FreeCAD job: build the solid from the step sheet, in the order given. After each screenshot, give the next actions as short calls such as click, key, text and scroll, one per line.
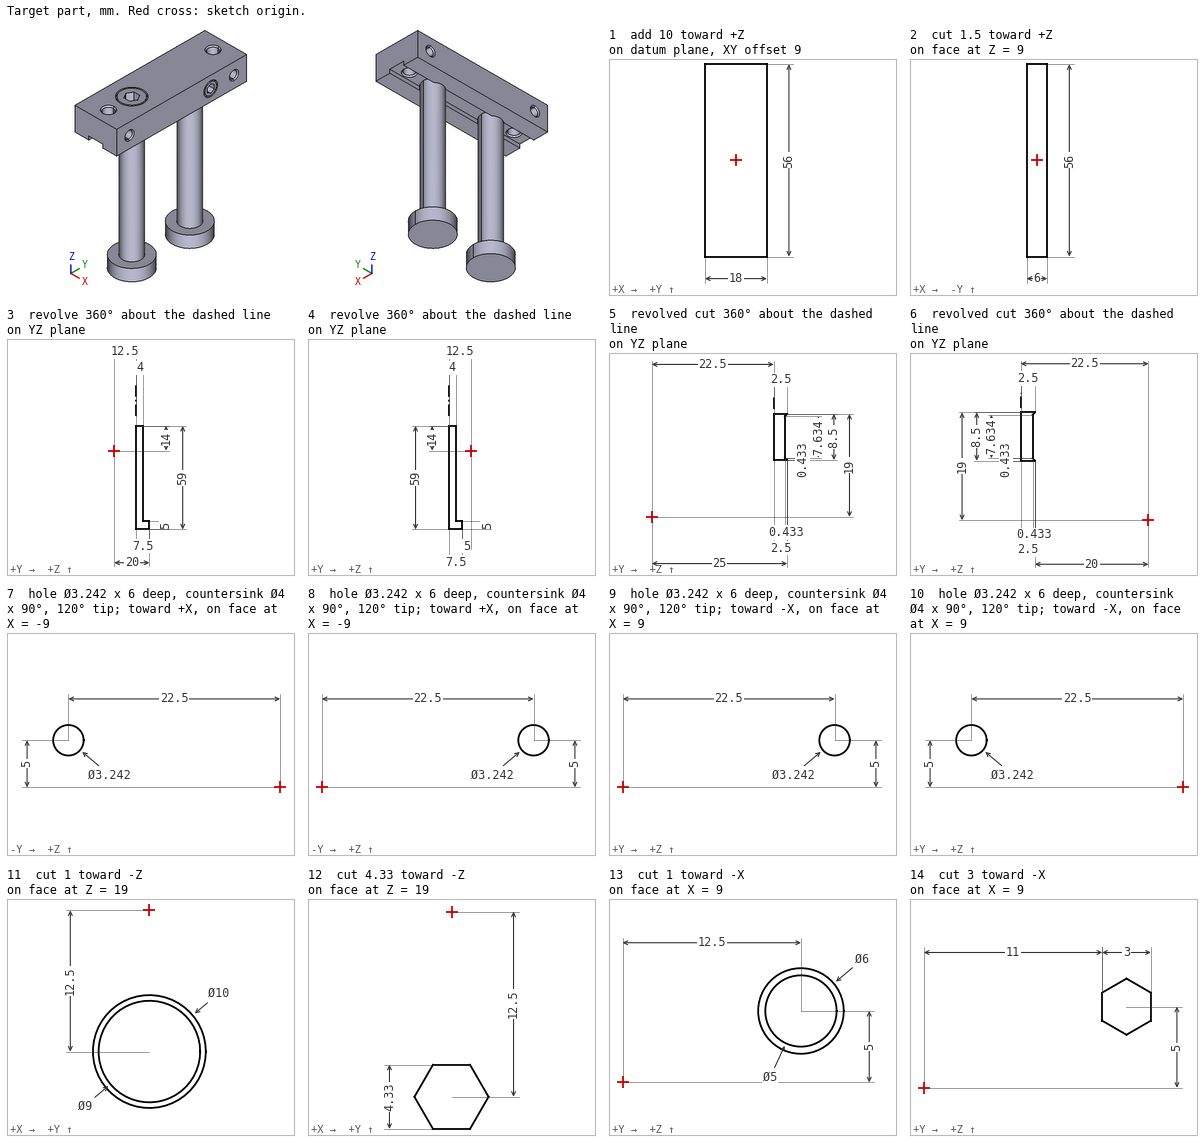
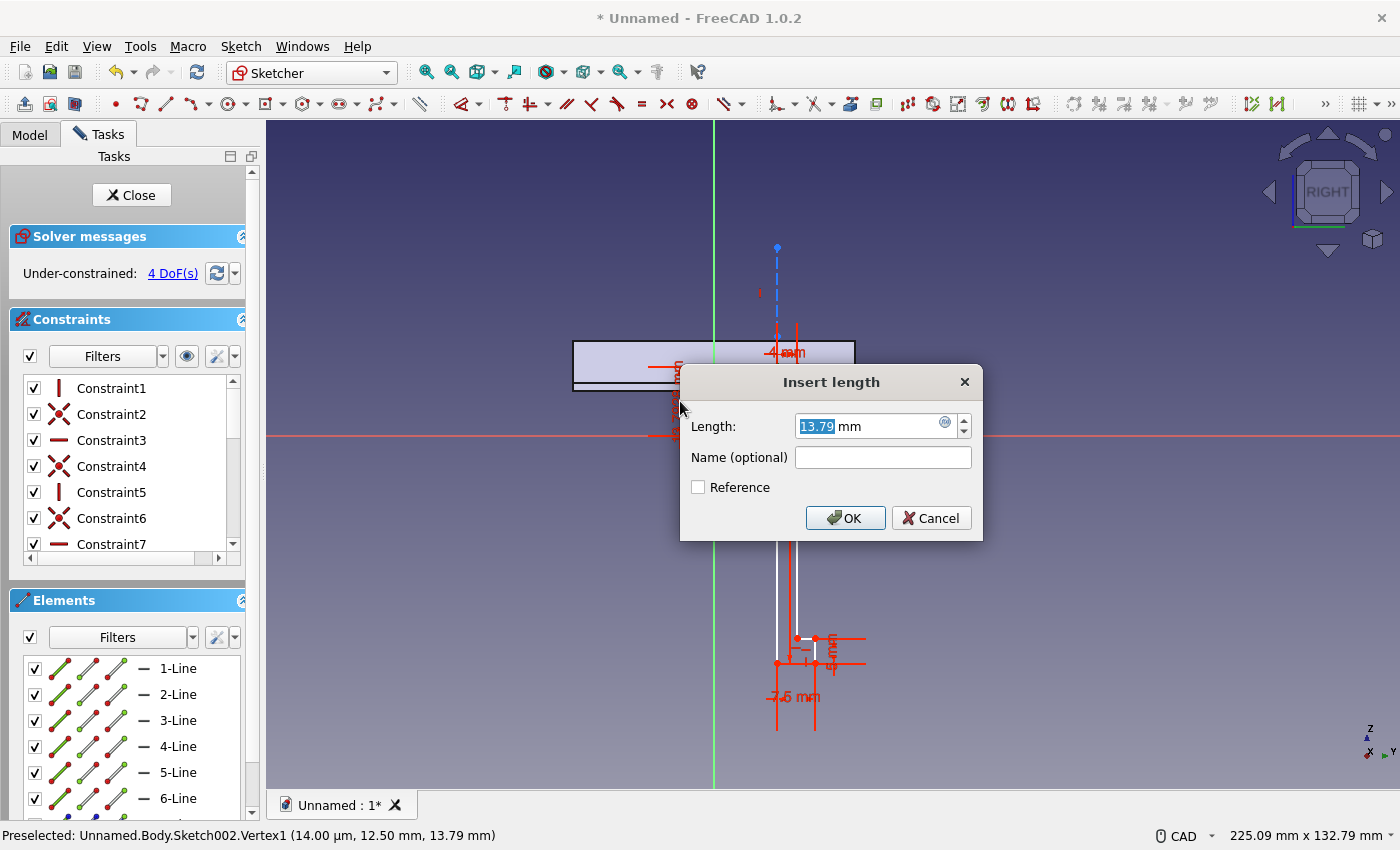
text(14)
key(Return)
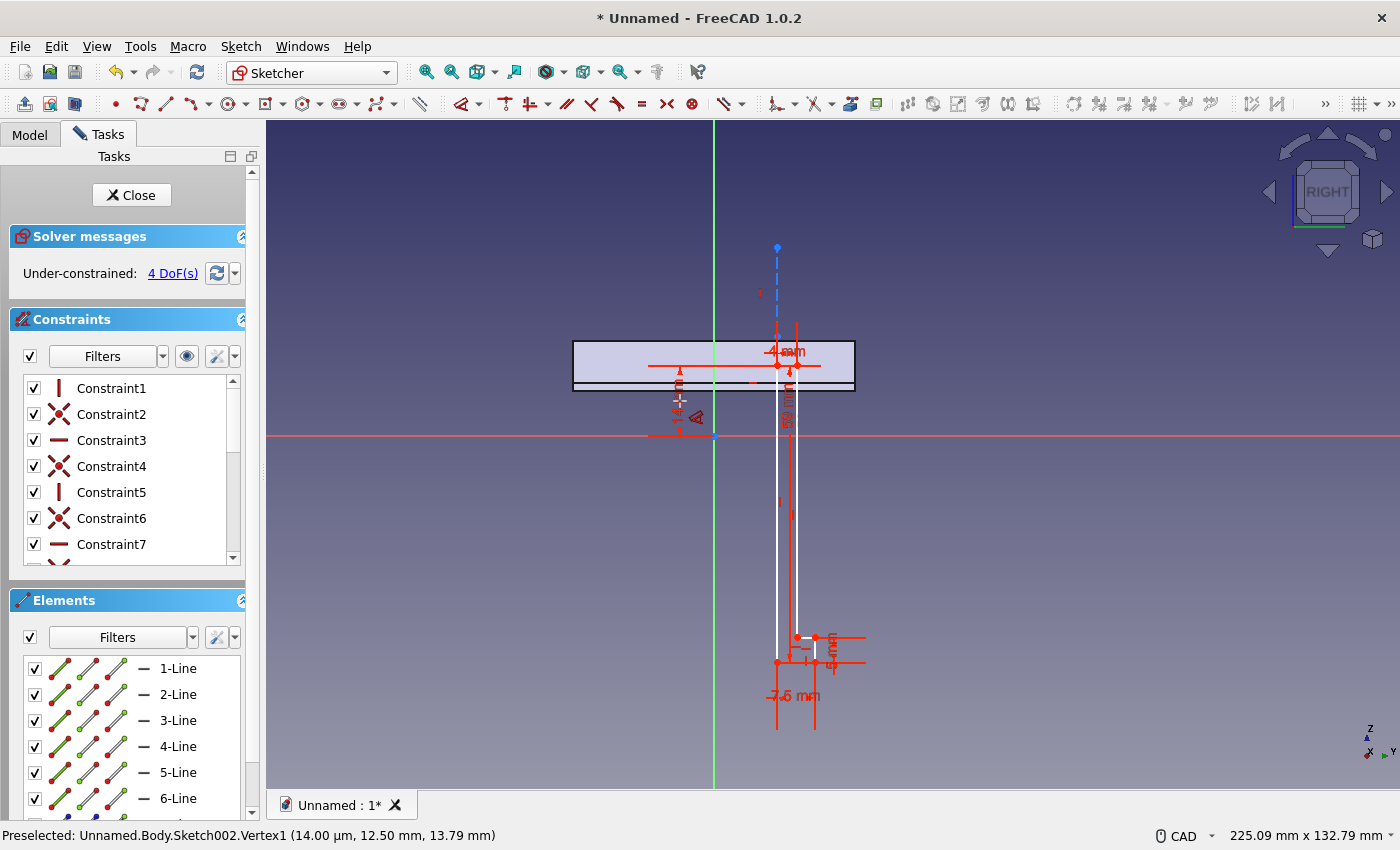
click(815, 663)
click(765, 721)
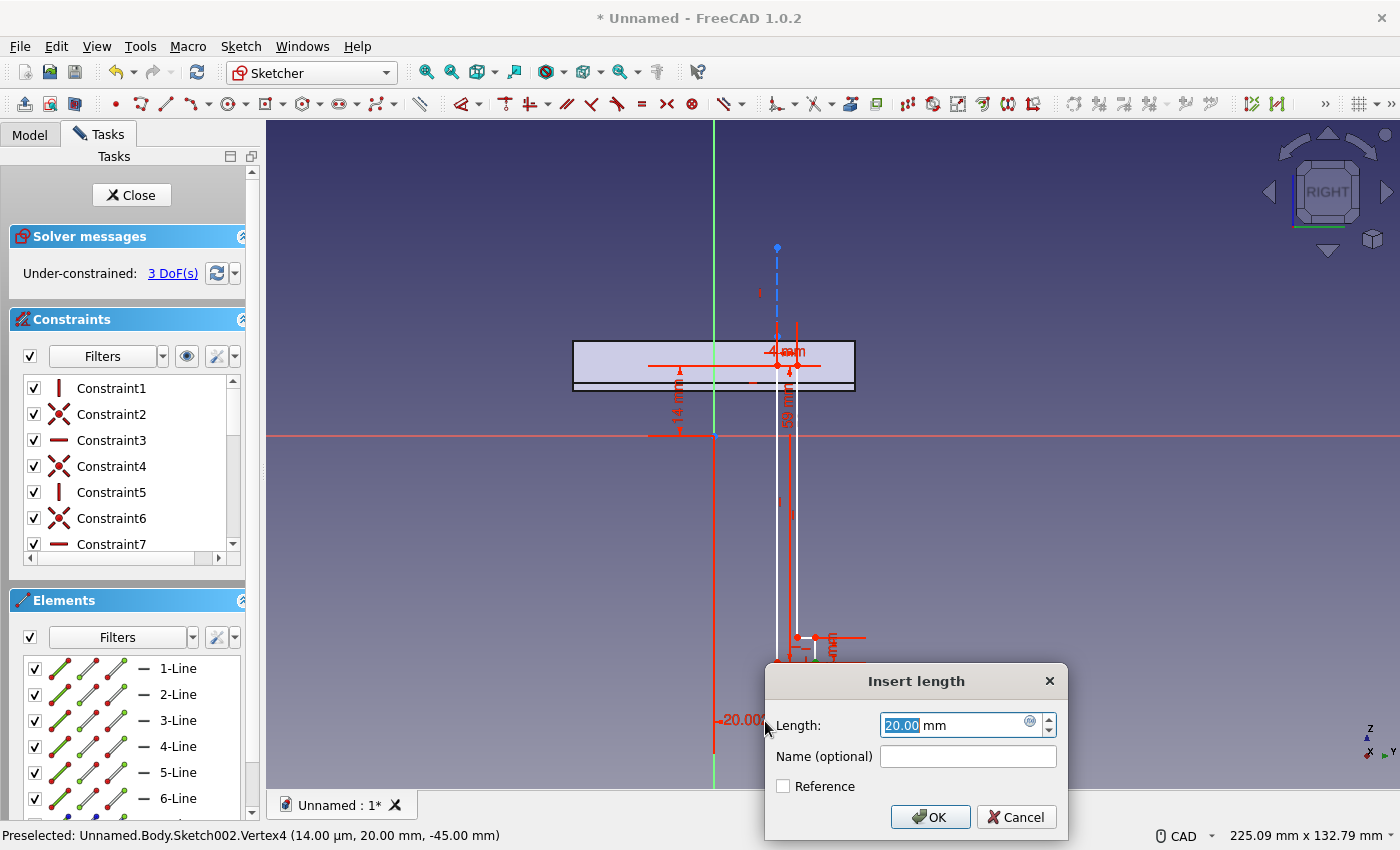
text(20)
key(Return)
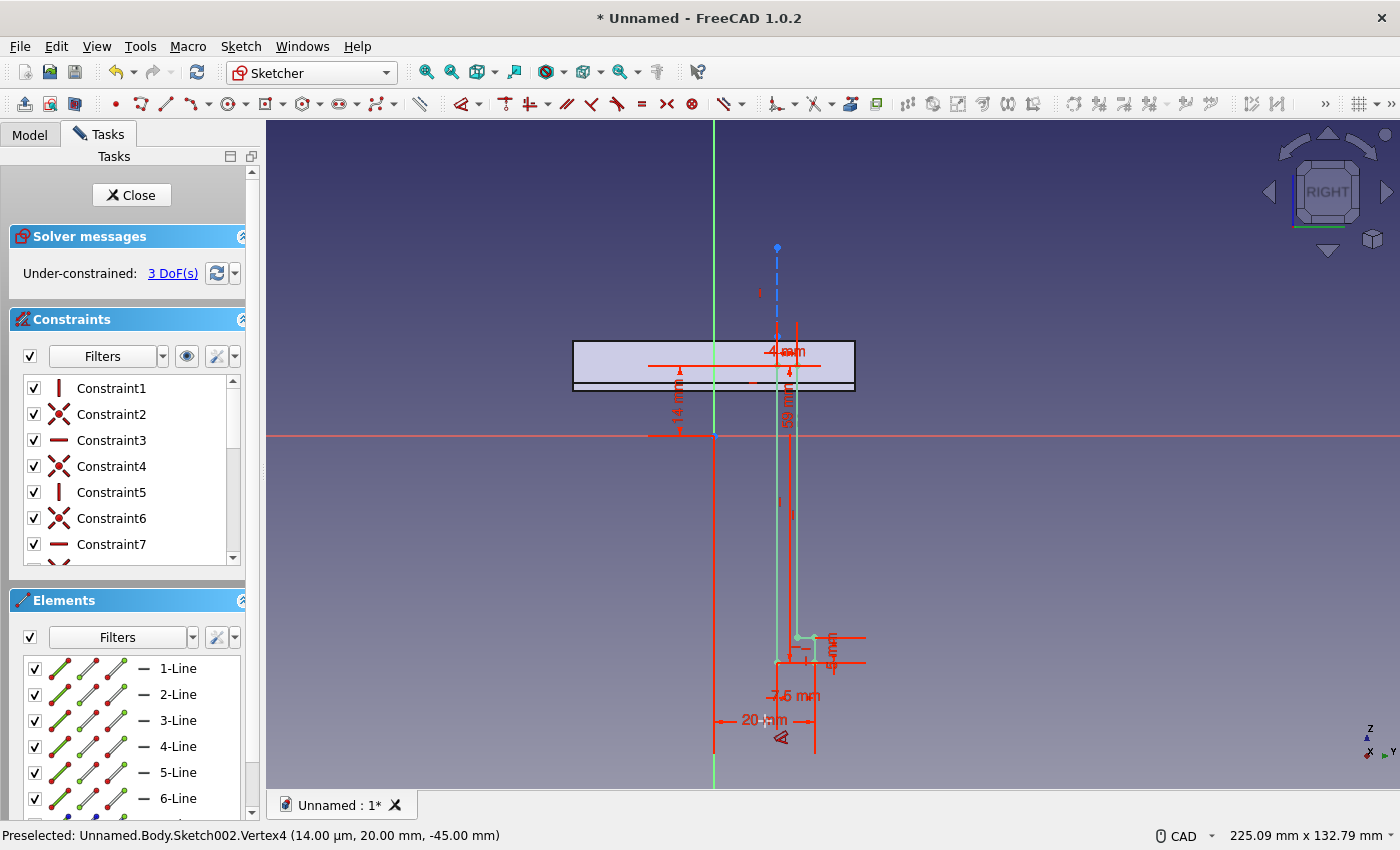
click(777, 337)
click(746, 303)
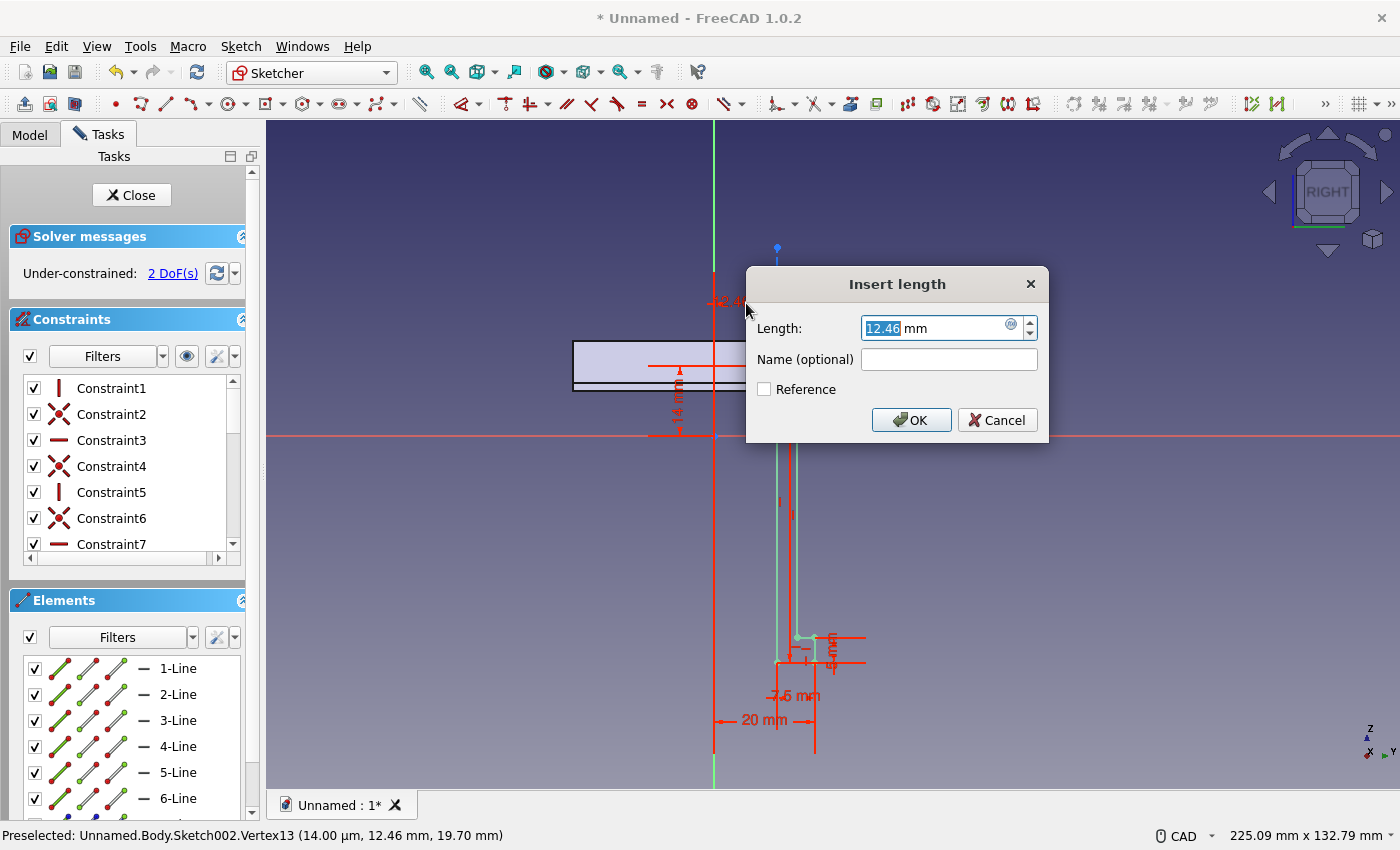
text(12.5)
key(Return)
key(Escape)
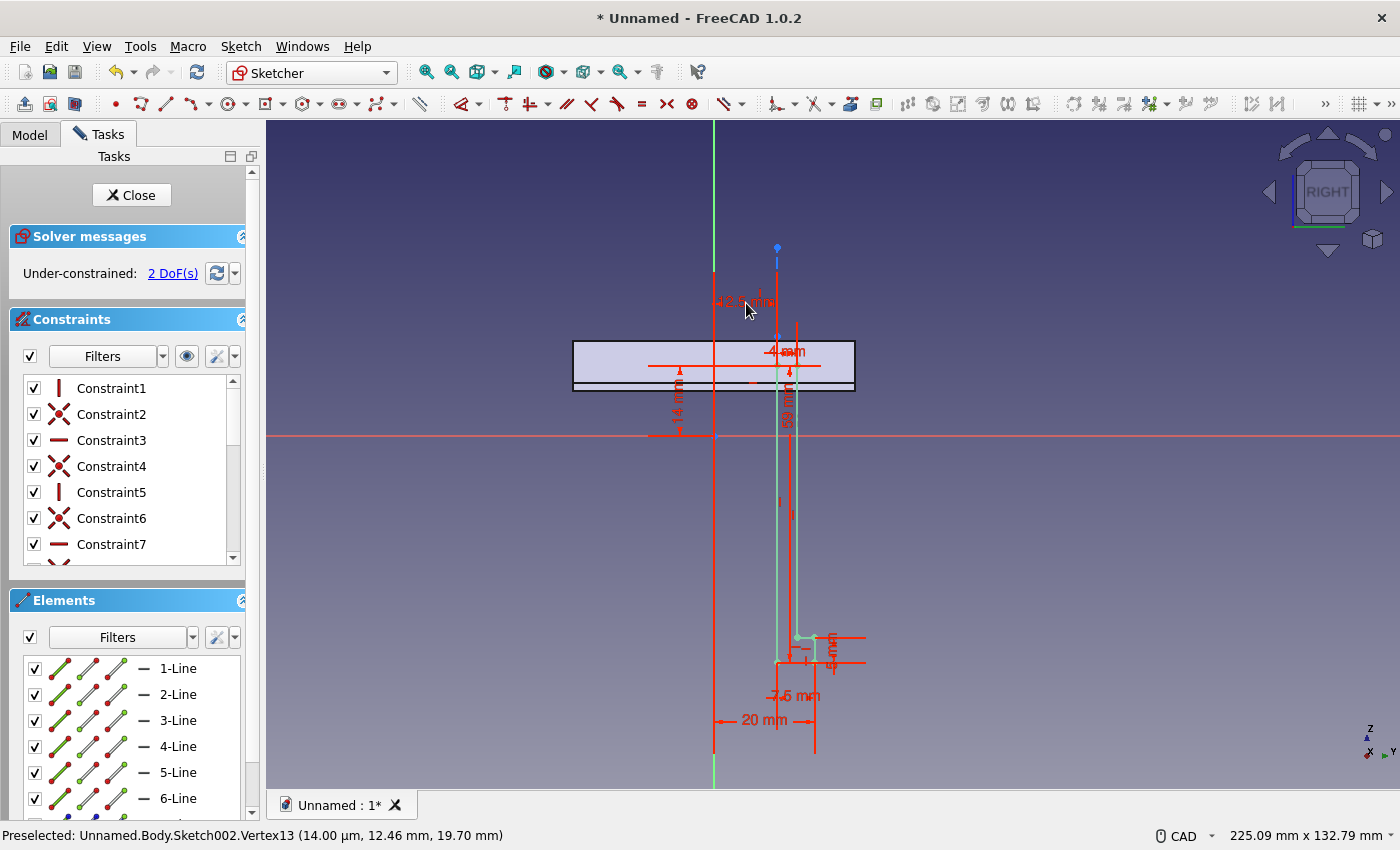
click(132, 195)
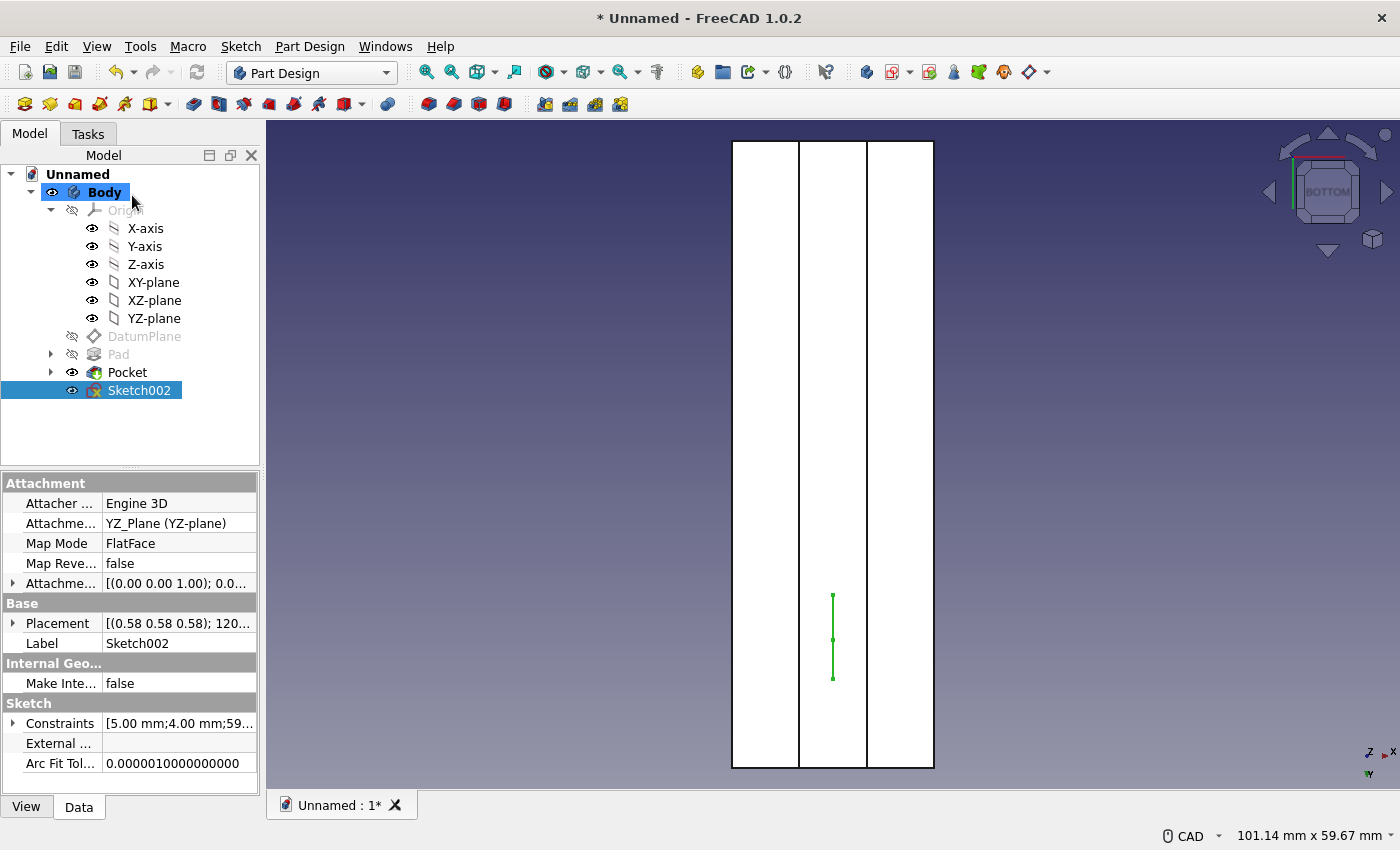
click(50, 104)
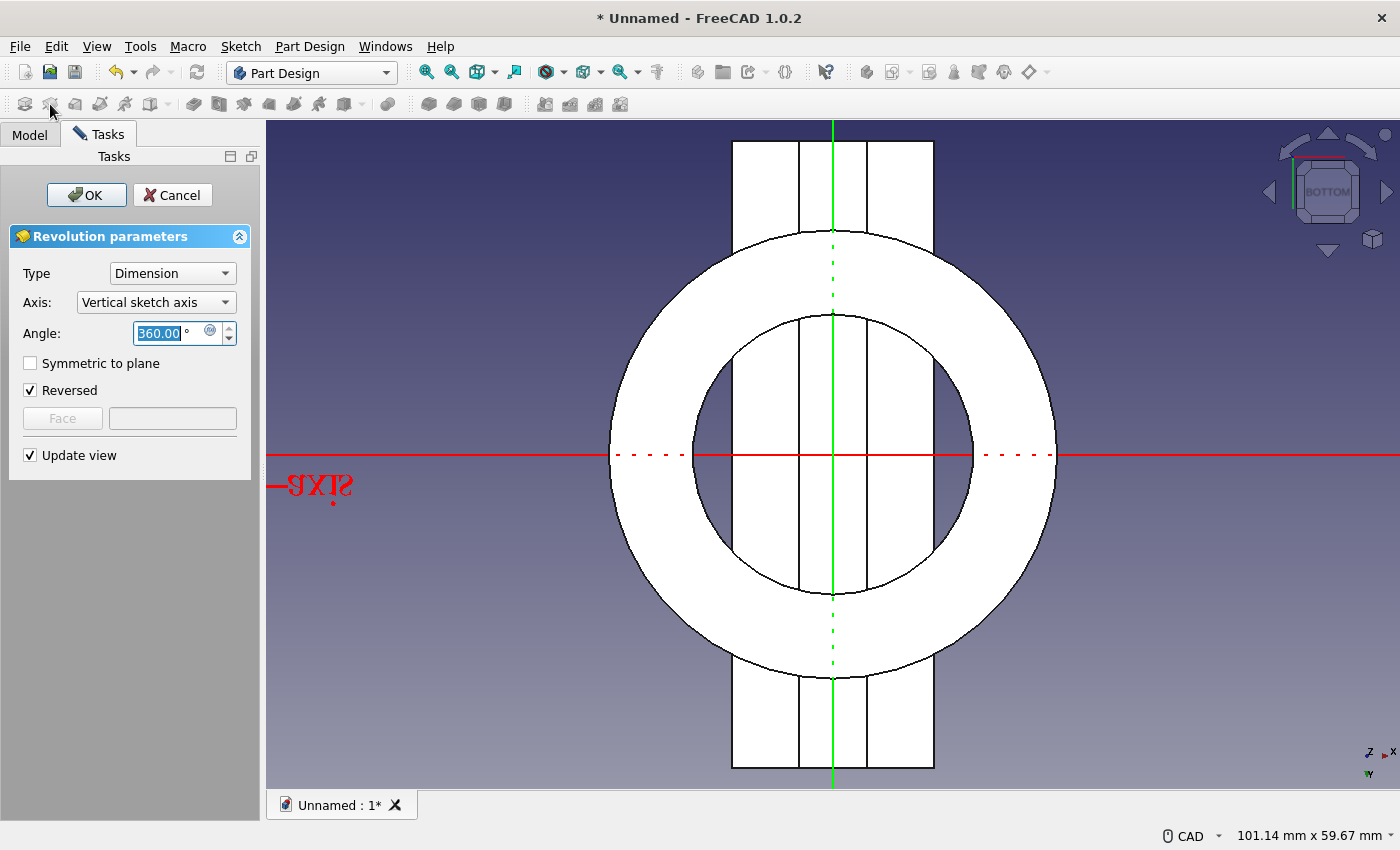
click(157, 302)